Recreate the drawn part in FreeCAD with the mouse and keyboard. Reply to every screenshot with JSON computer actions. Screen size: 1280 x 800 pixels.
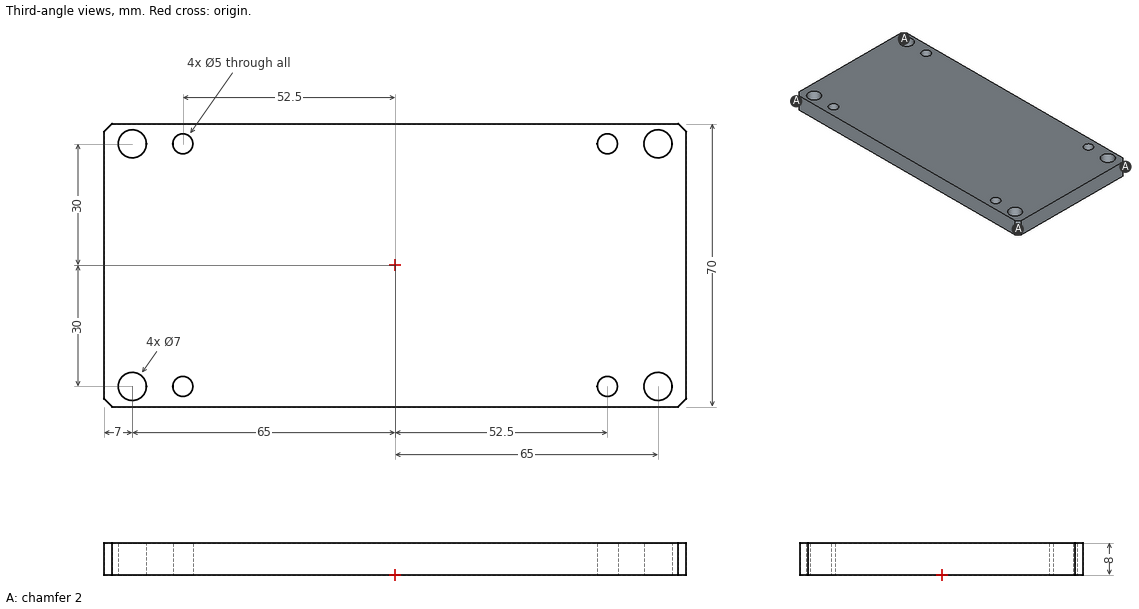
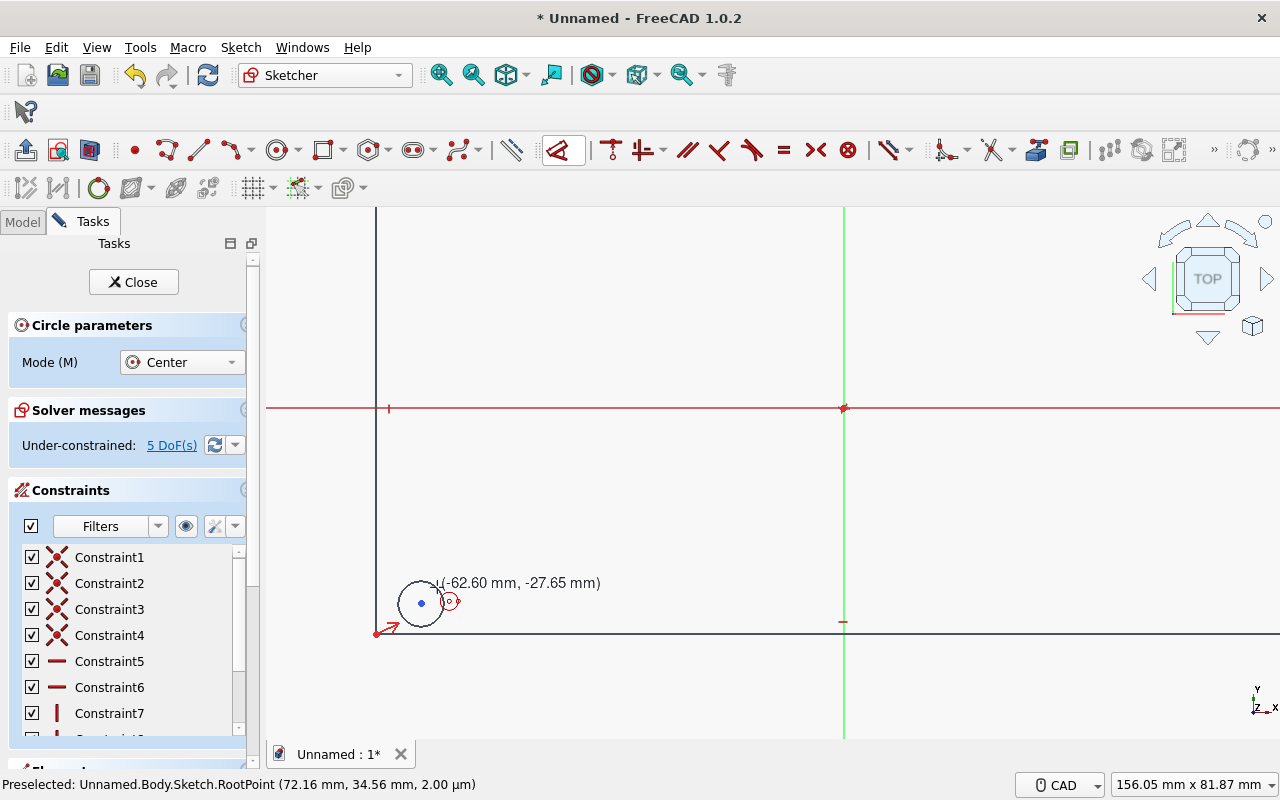
{"action": "scroll", "coordinate": [421, 604], "scroll_direction": "down", "scroll_amount": 2}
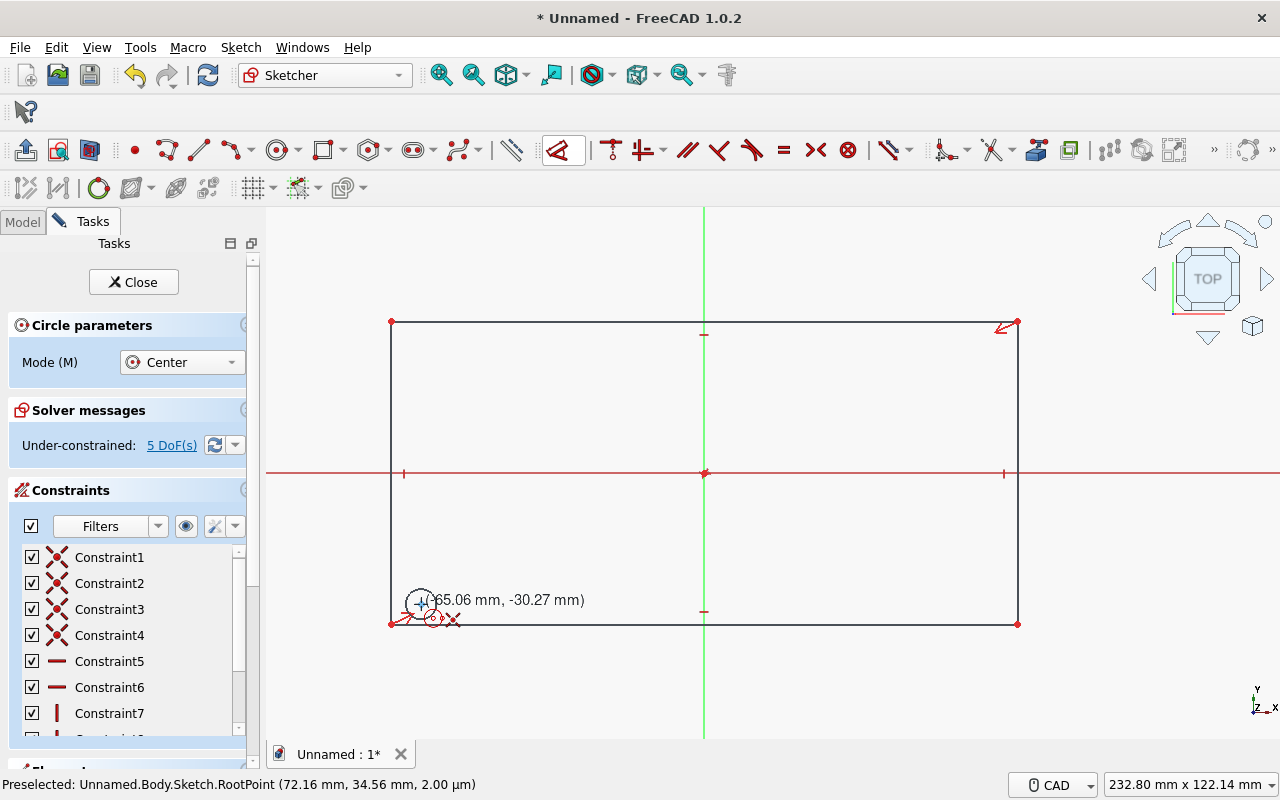
{"action": "scroll", "coordinate": [988, 604], "scroll_direction": "up", "scroll_amount": 2}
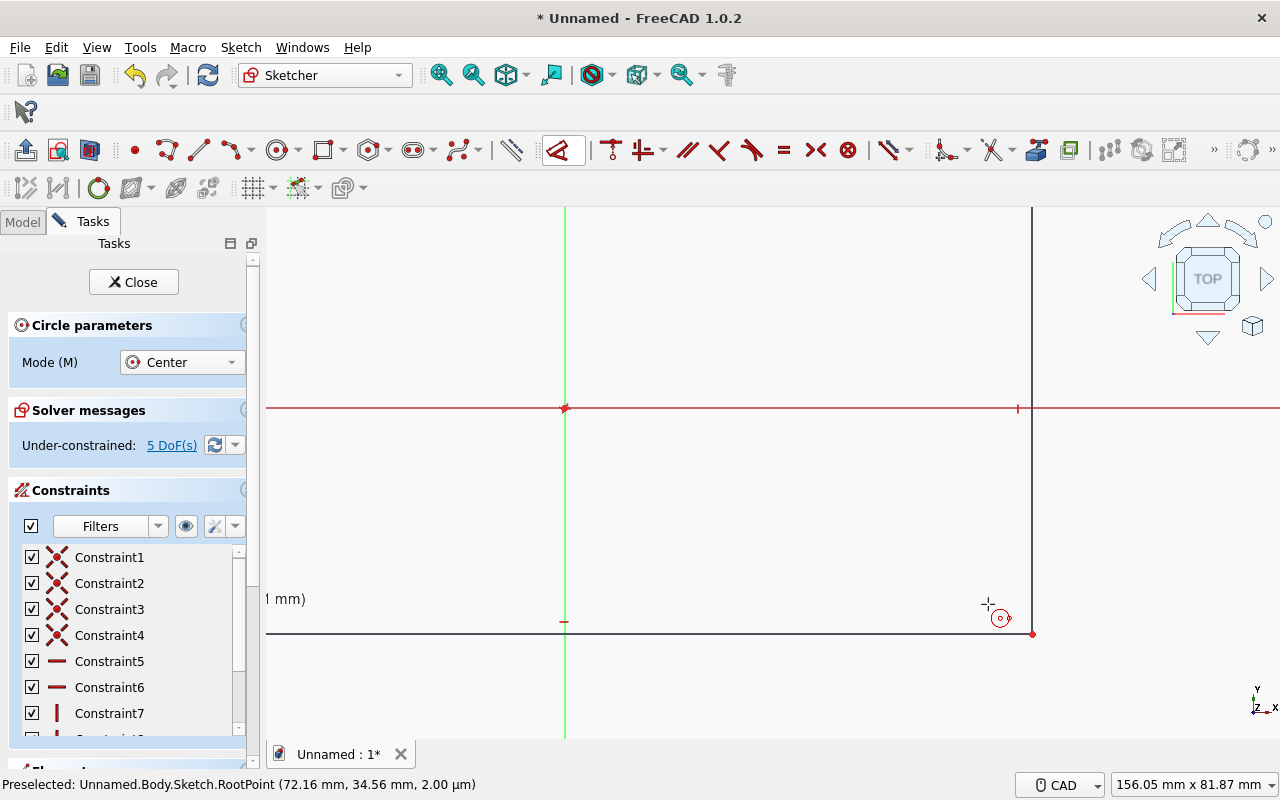
{"action": "left_click", "coordinate": [987, 603]}
{"action": "left_click", "coordinate": [1003, 587]}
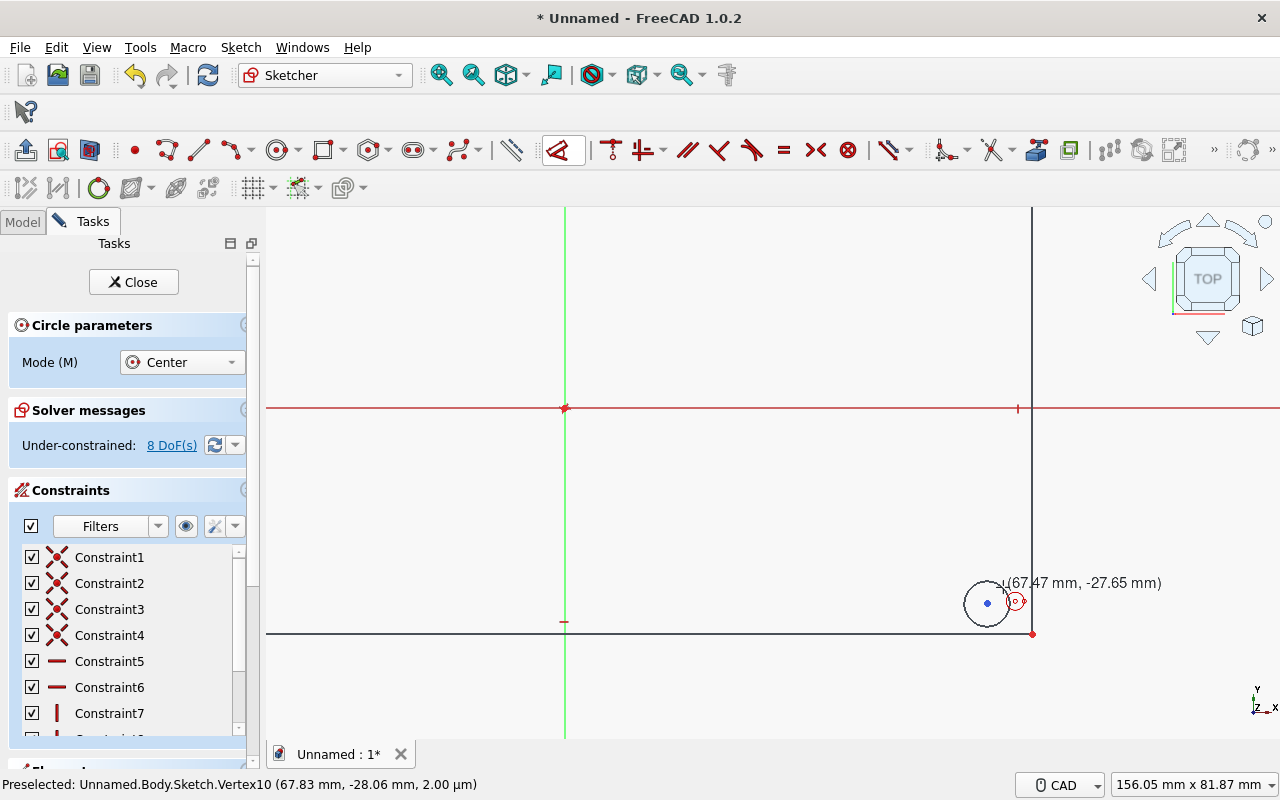
{"action": "scroll", "coordinate": [989, 604], "scroll_direction": "down", "scroll_amount": 2}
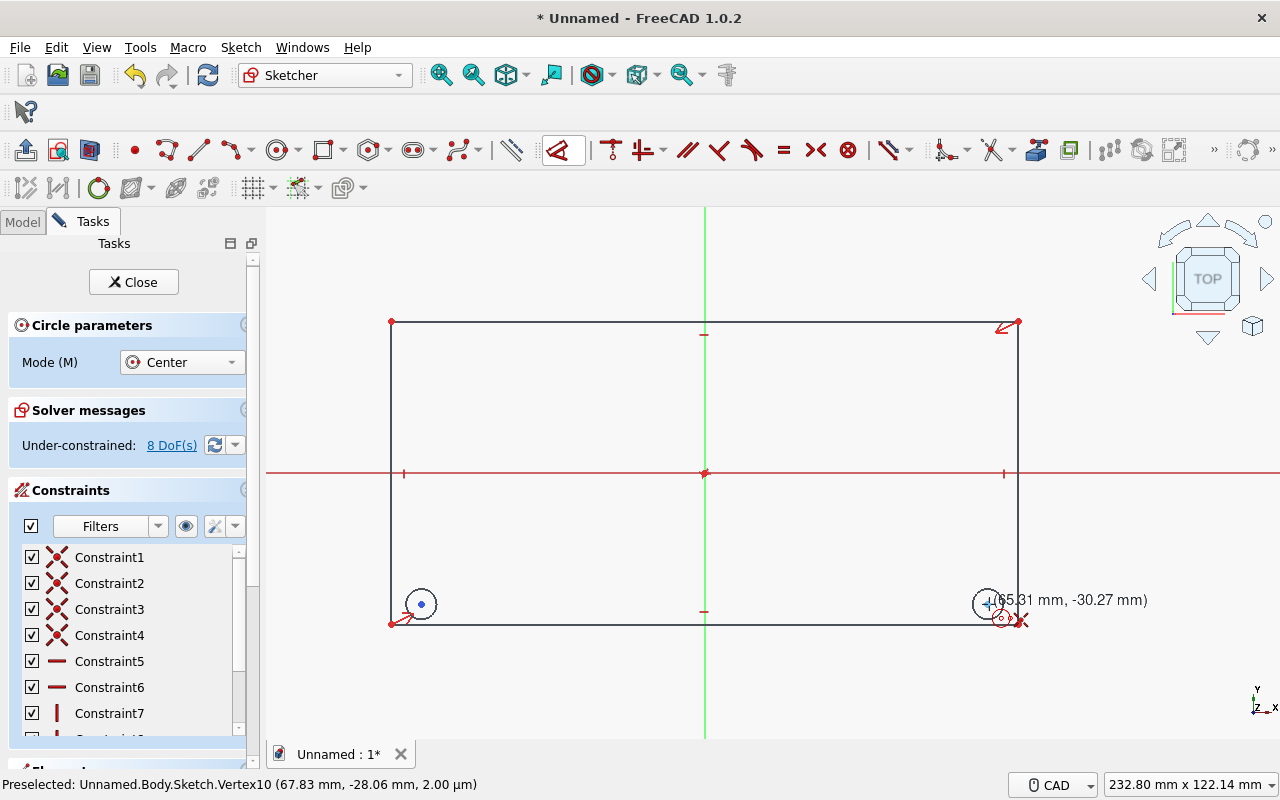
{"action": "scroll", "coordinate": [422, 342], "scroll_direction": "up", "scroll_amount": 2}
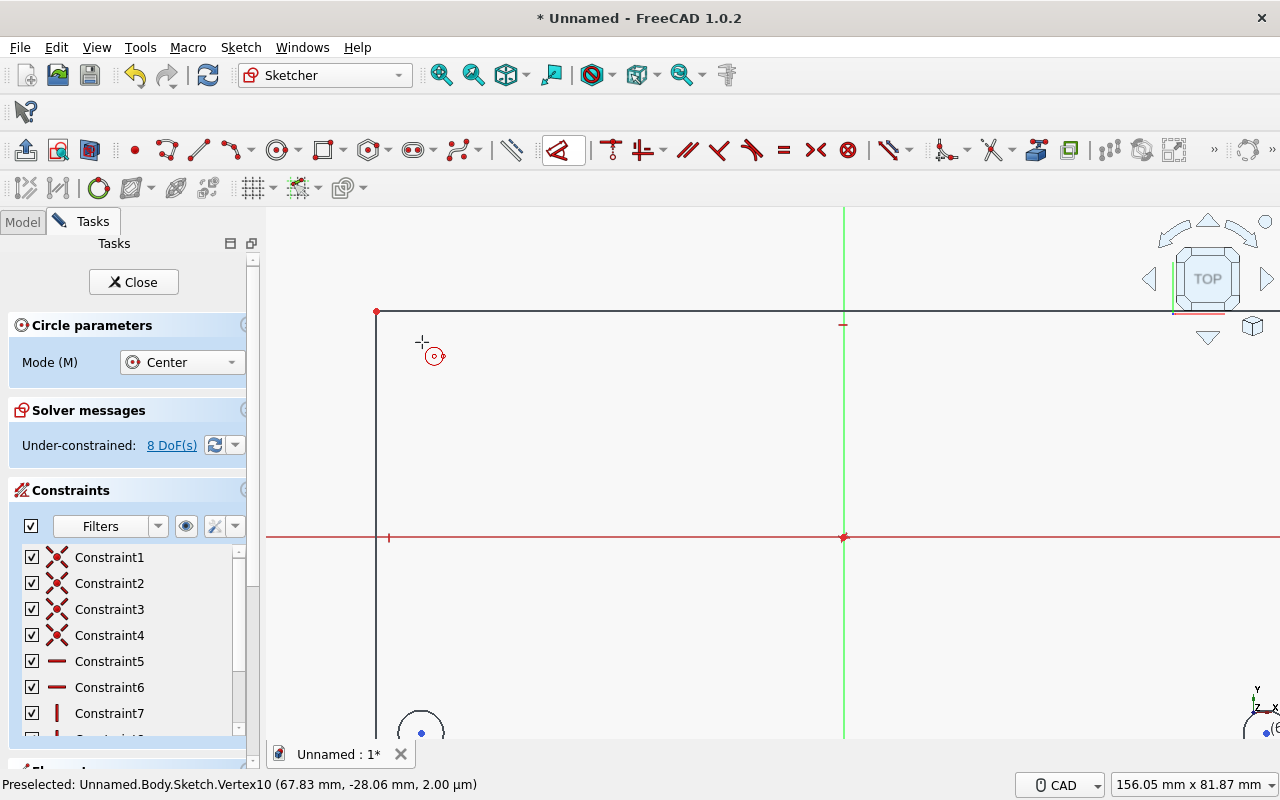
{"action": "left_click", "coordinate": [421, 343]}
{"action": "left_click", "coordinate": [437, 326]}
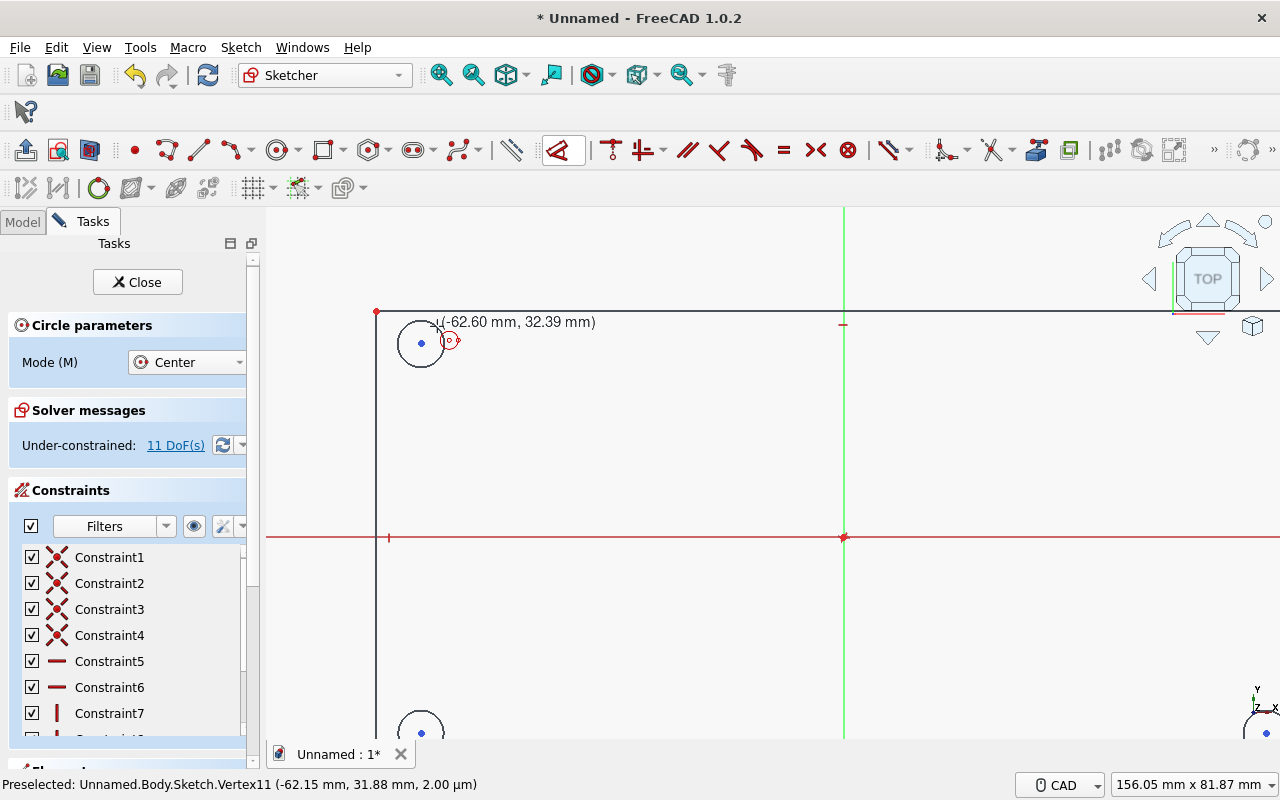
{"action": "scroll", "coordinate": [421, 342], "scroll_direction": "down", "scroll_amount": 2}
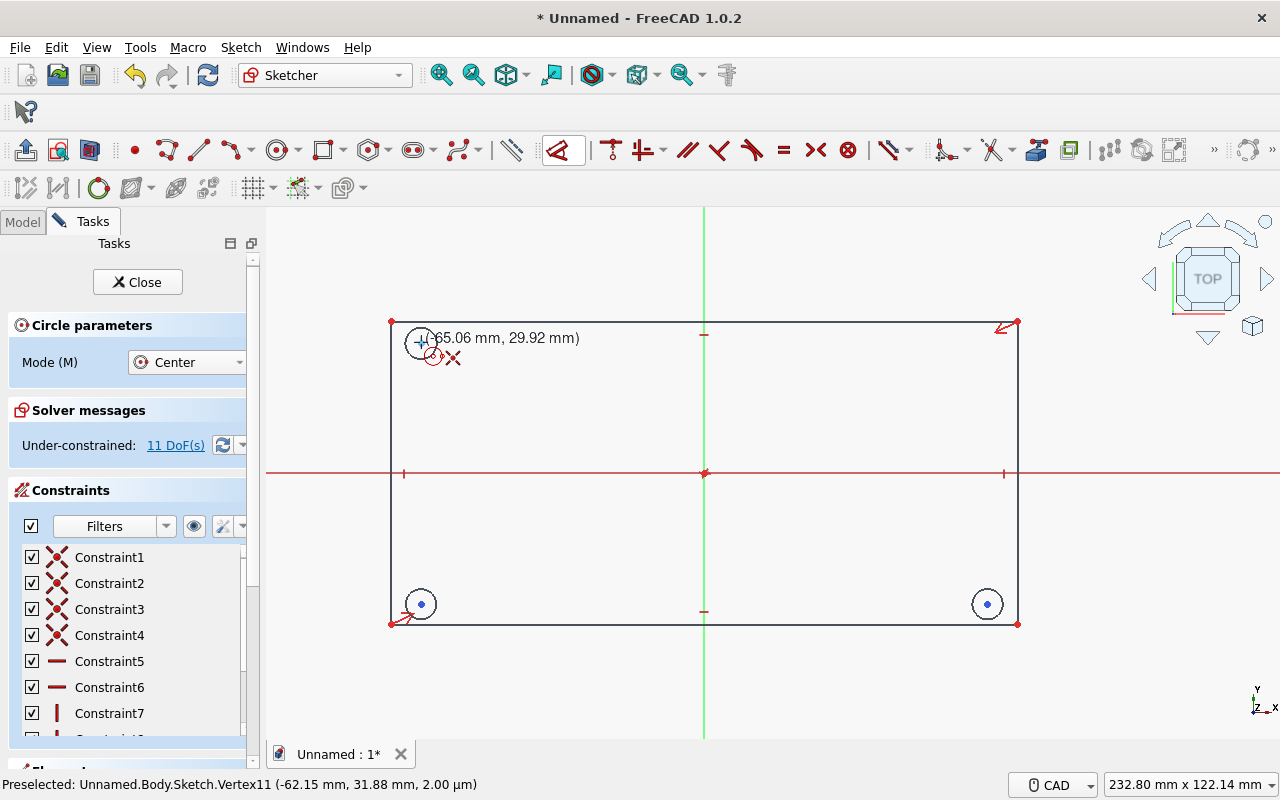
{"action": "scroll", "coordinate": [988, 342], "scroll_direction": "up", "scroll_amount": 2}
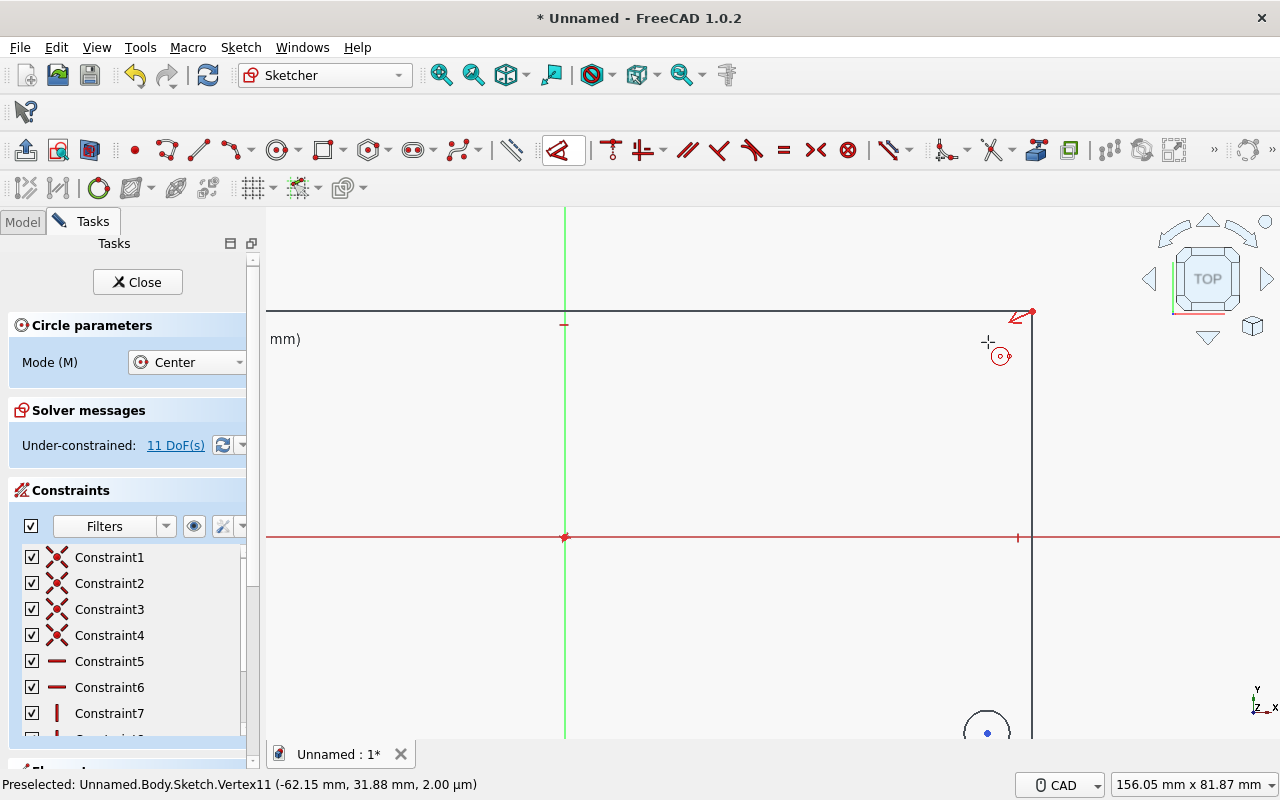
{"action": "left_click", "coordinate": [987, 343]}
{"action": "left_click", "coordinate": [1003, 326]}
{"action": "key", "text": "Escape"}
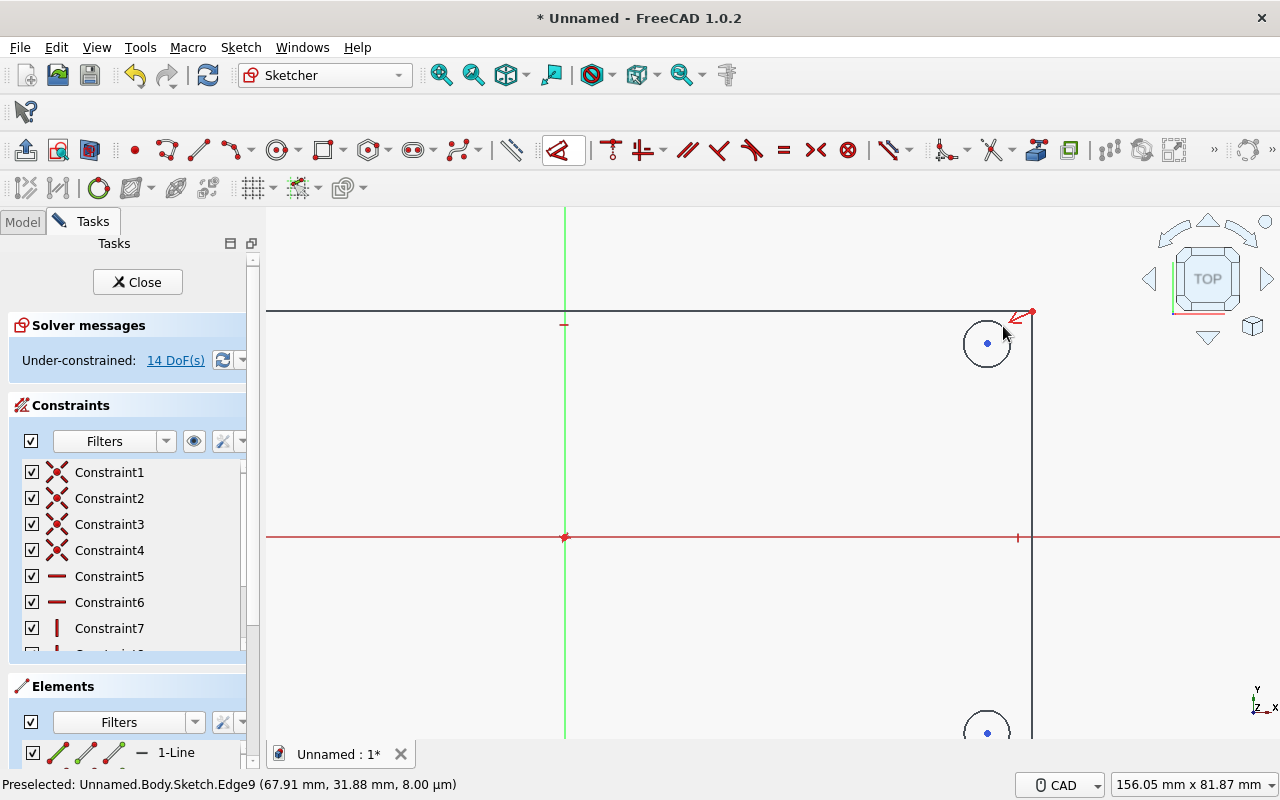
{"action": "scroll", "coordinate": [989, 342], "scroll_direction": "down", "scroll_amount": 2}